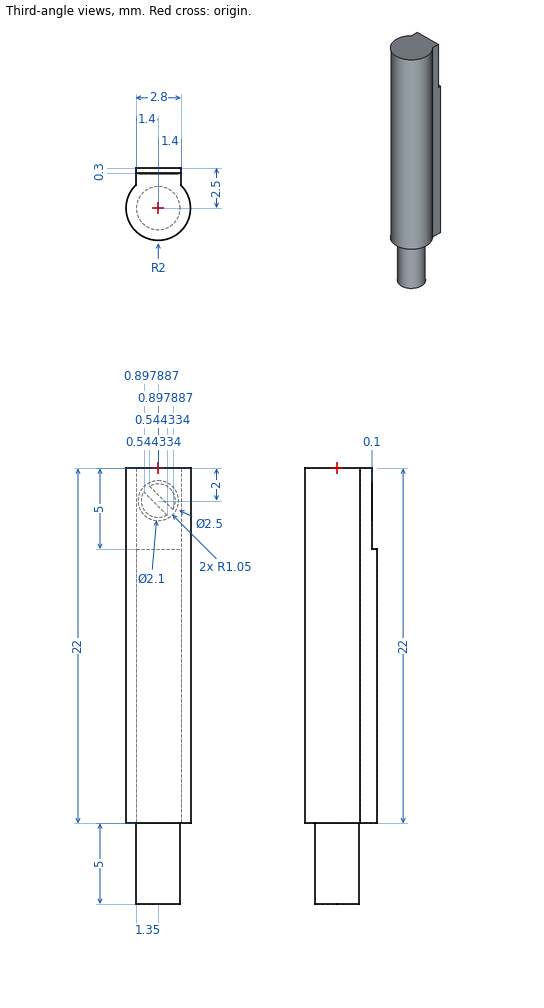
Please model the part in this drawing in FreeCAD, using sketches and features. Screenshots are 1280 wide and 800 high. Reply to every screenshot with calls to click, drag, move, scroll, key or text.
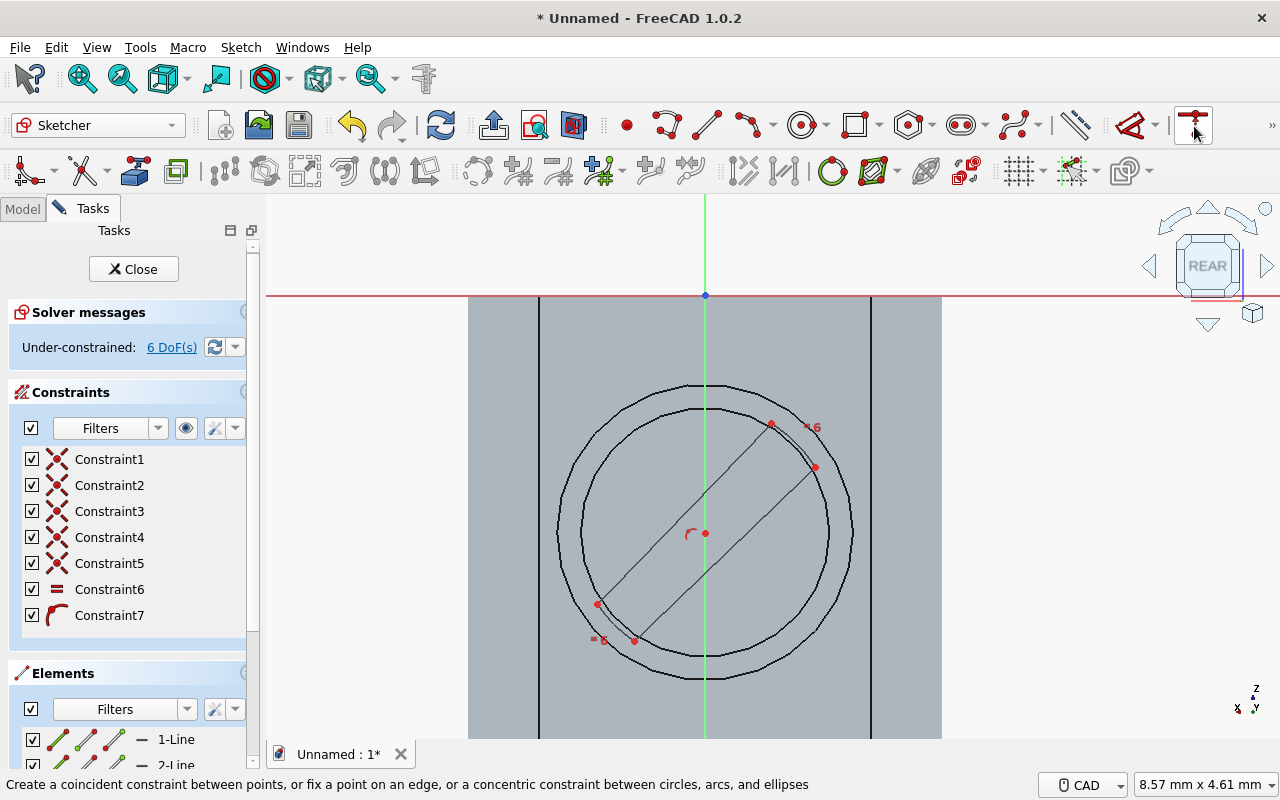
click(1130, 126)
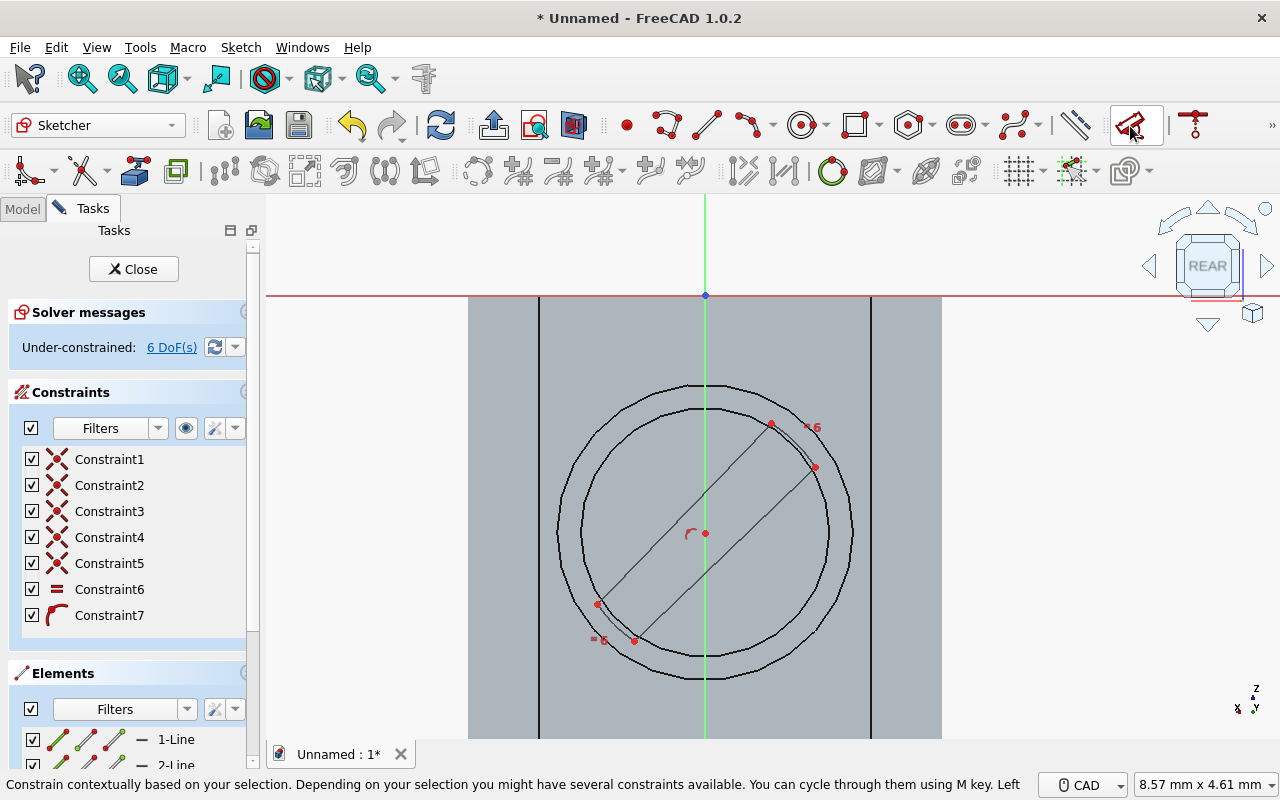
click(607, 617)
click(583, 638)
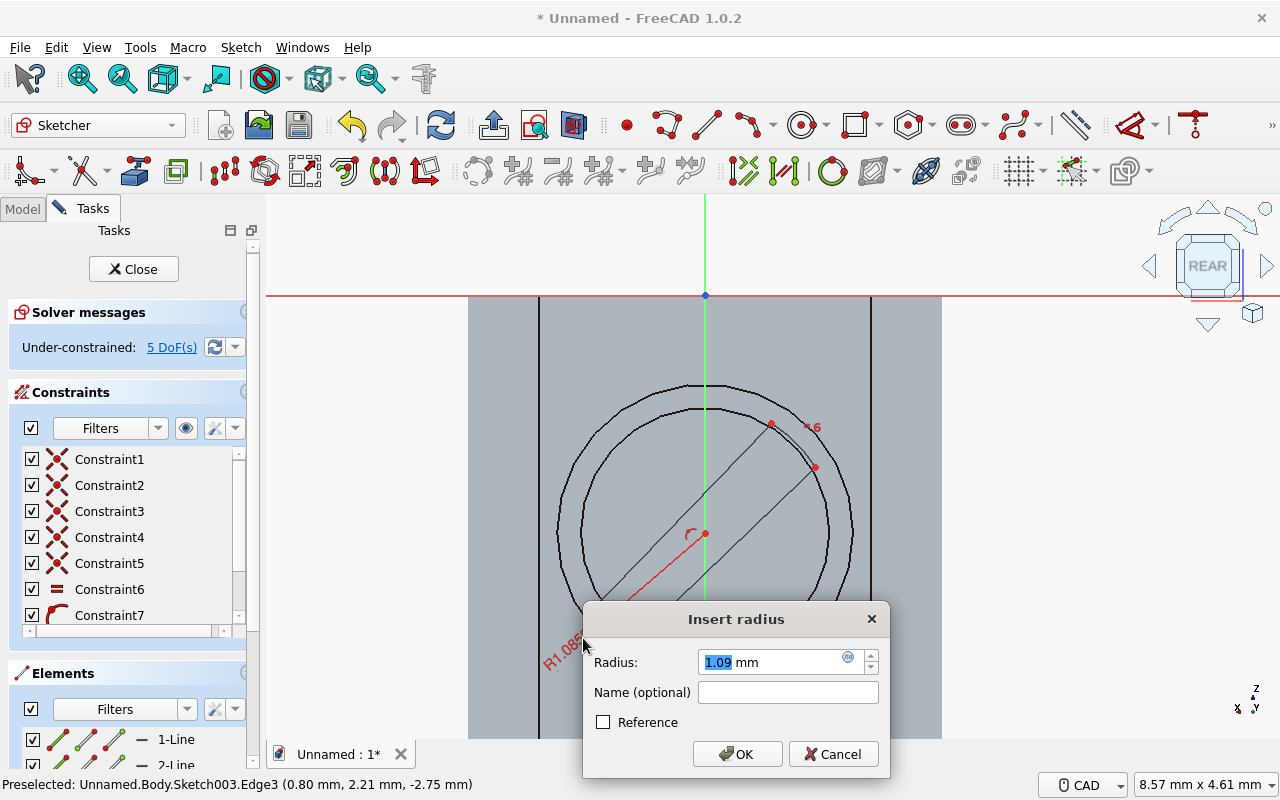
text(1.05)
key(Return)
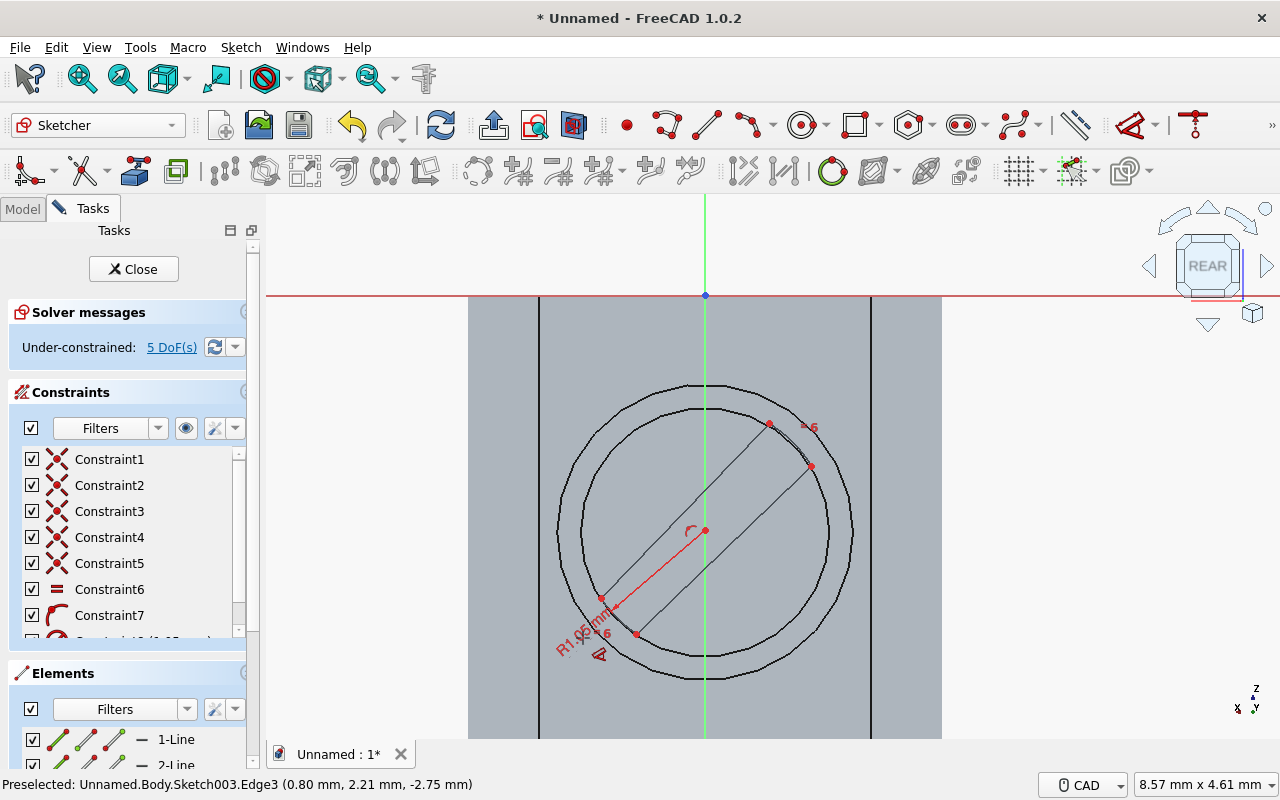
click(705, 530)
click(739, 413)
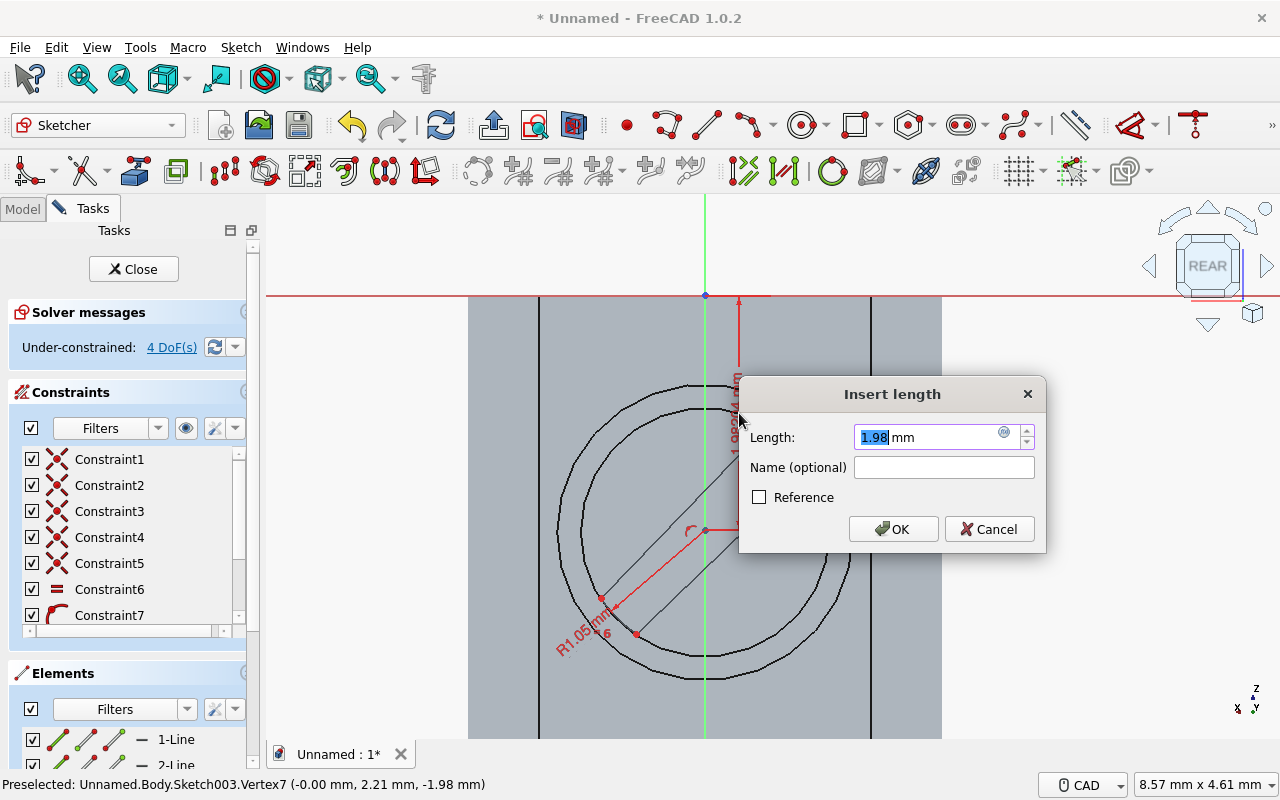
text(2)
key(Return)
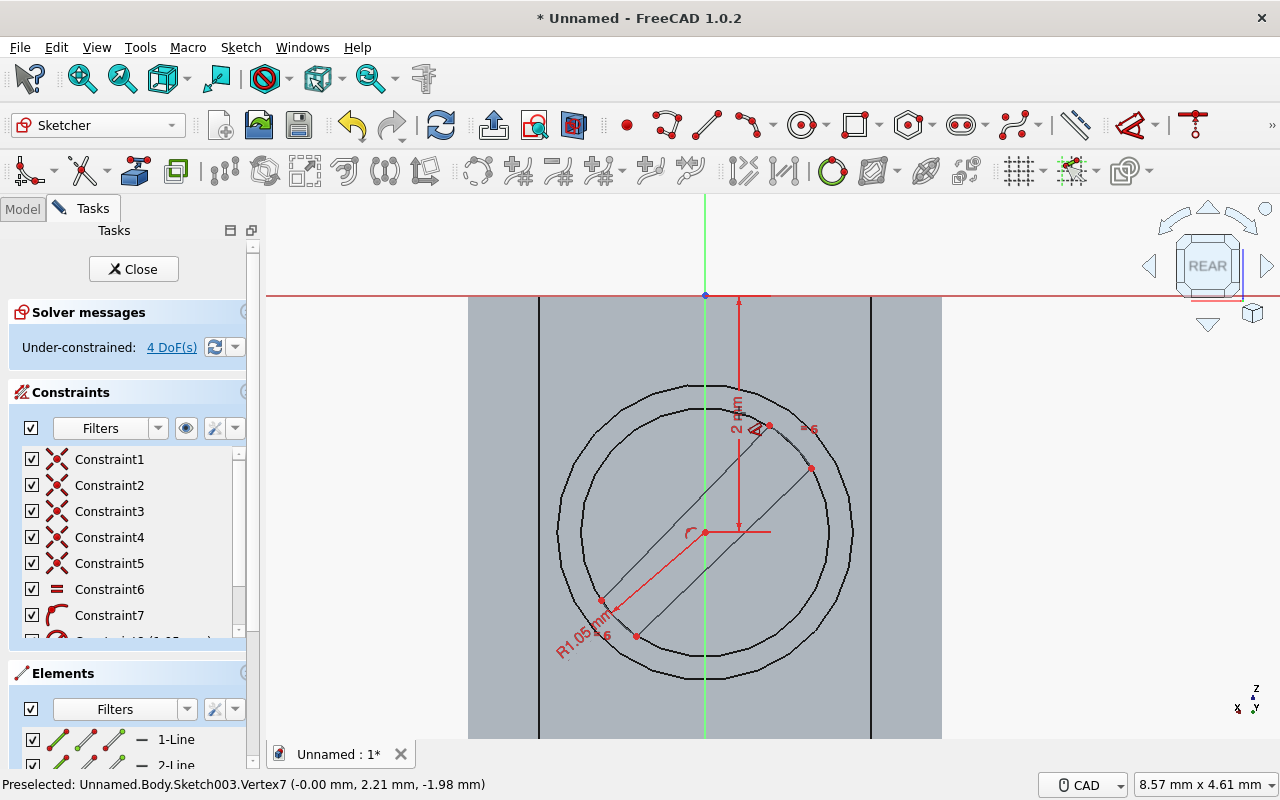
click(769, 426)
click(737, 262)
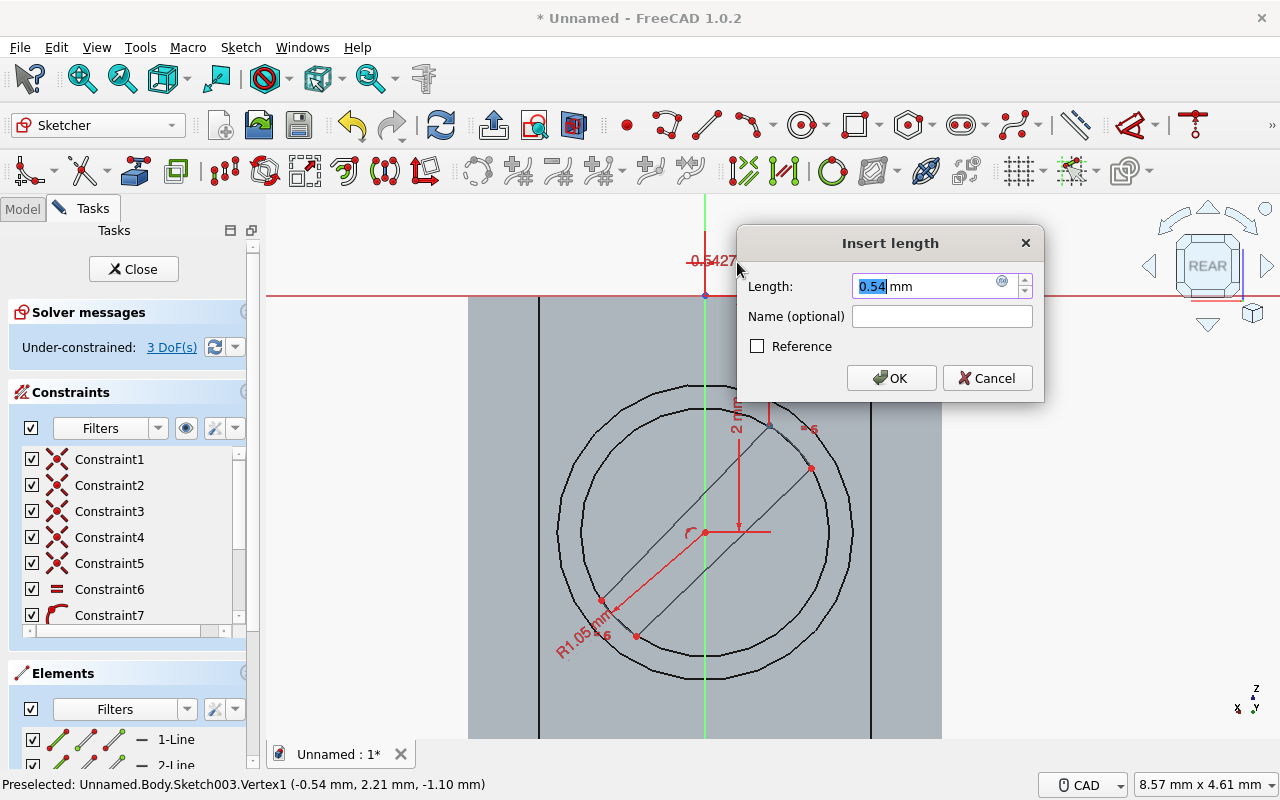
text(0.544334)
key(Return)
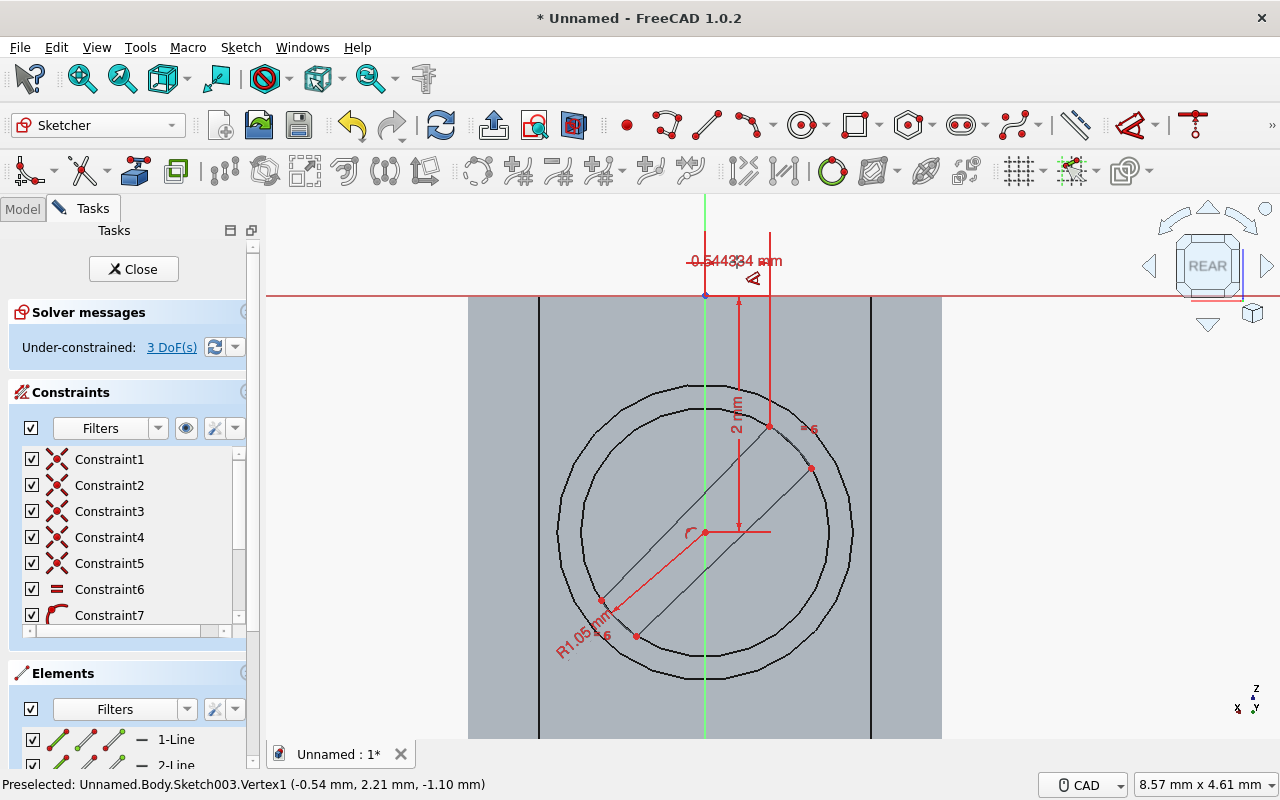
click(601, 601)
click(653, 262)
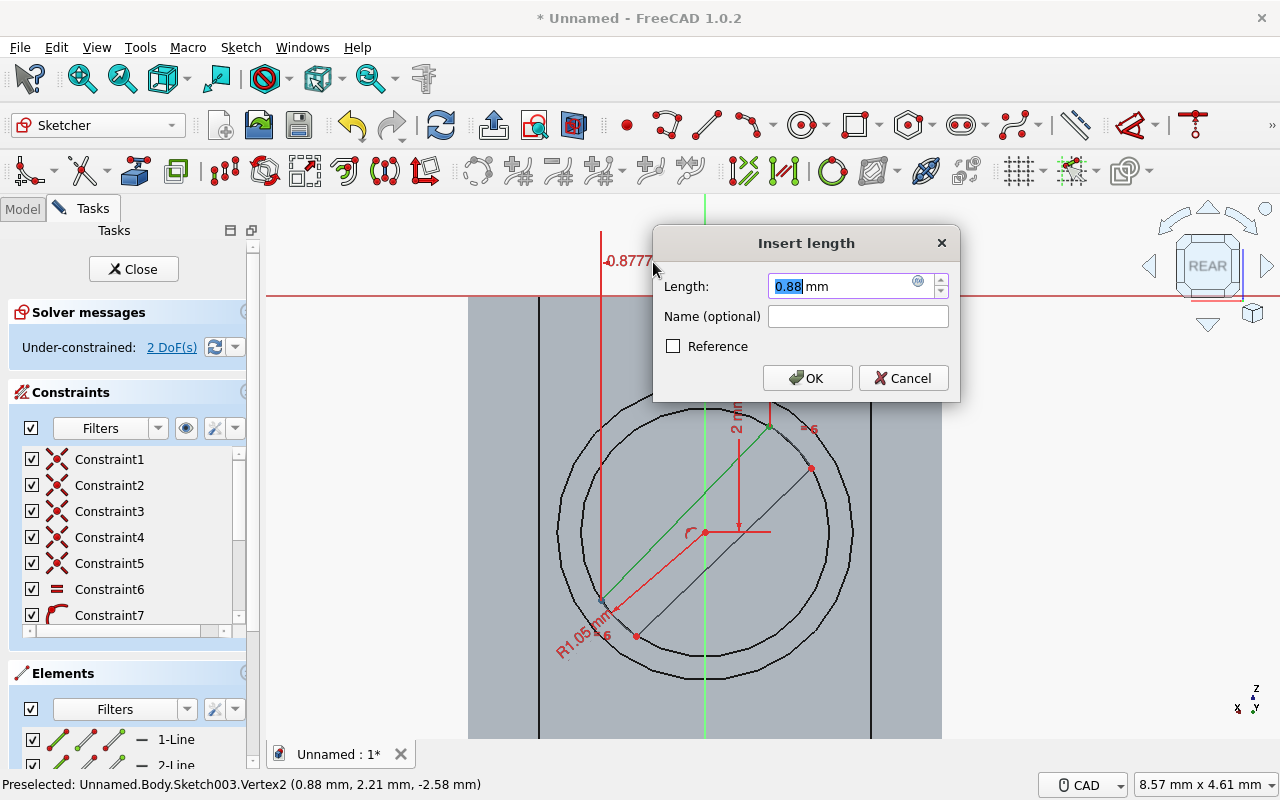
text(0.897887)
key(Return)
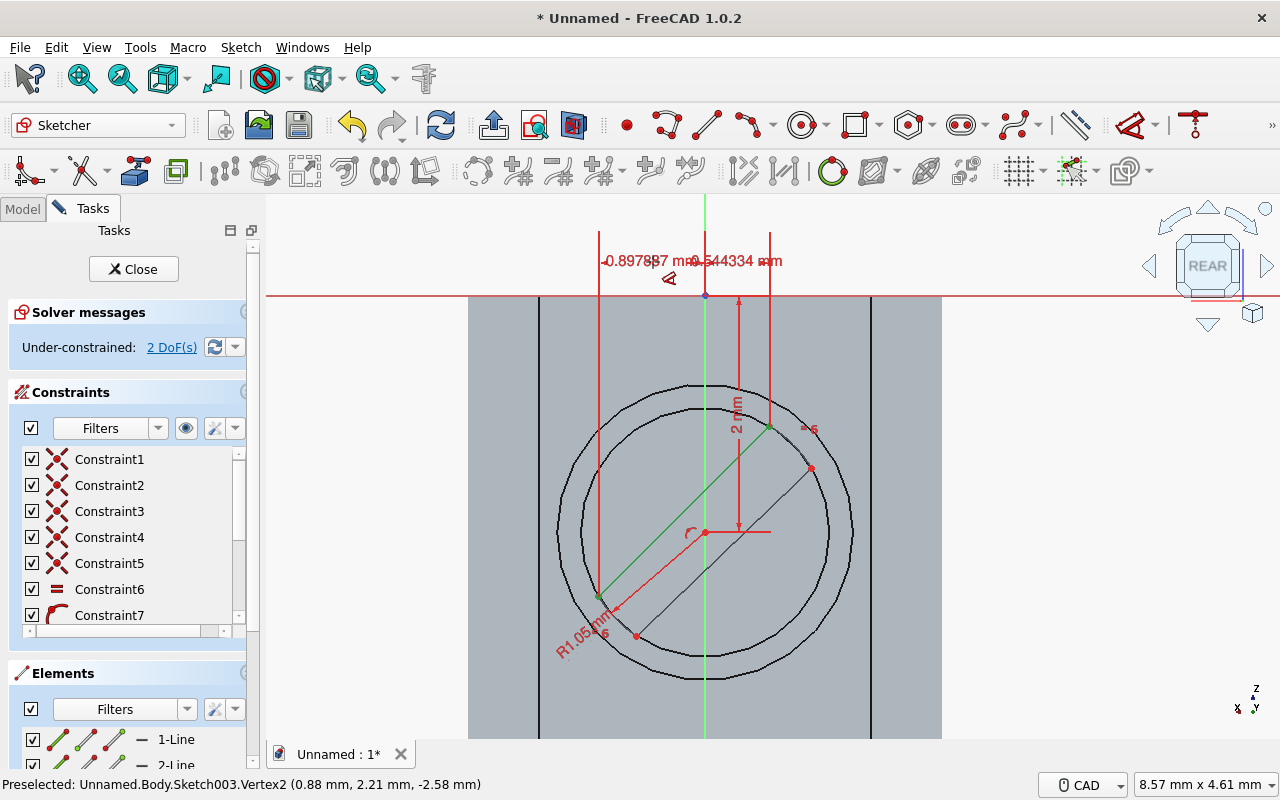
click(637, 636)
click(671, 670)